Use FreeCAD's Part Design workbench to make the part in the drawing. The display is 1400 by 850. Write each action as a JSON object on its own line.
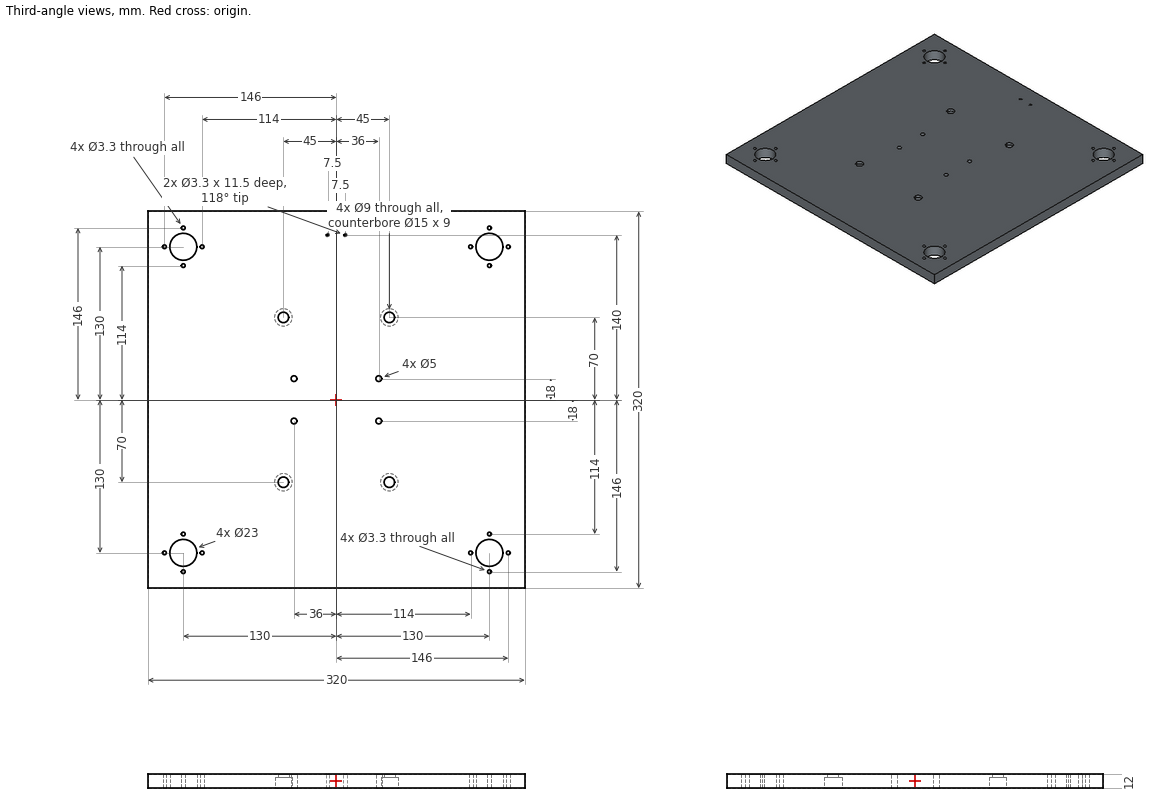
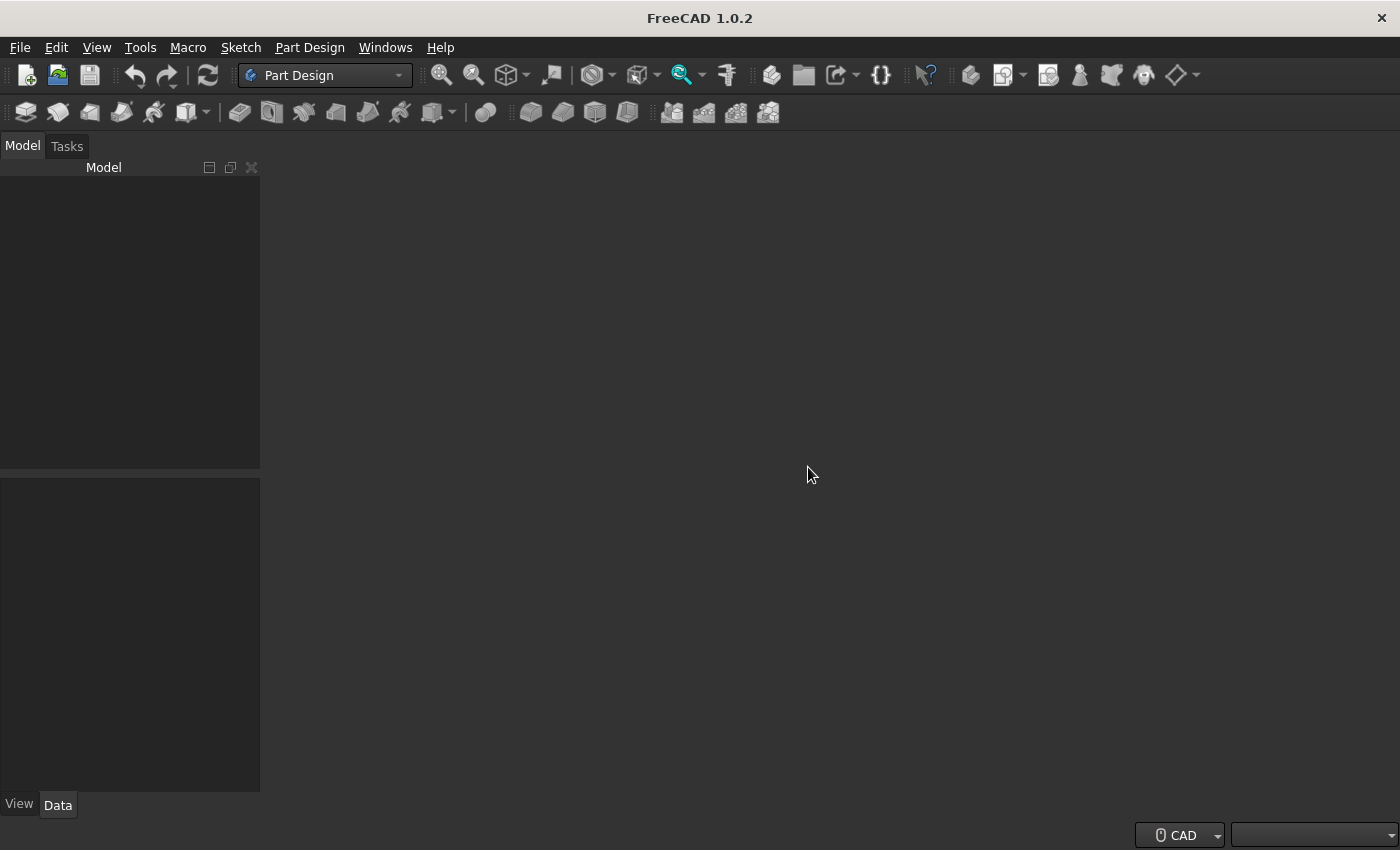
{"action": "left_click", "coordinate": [26, 76]}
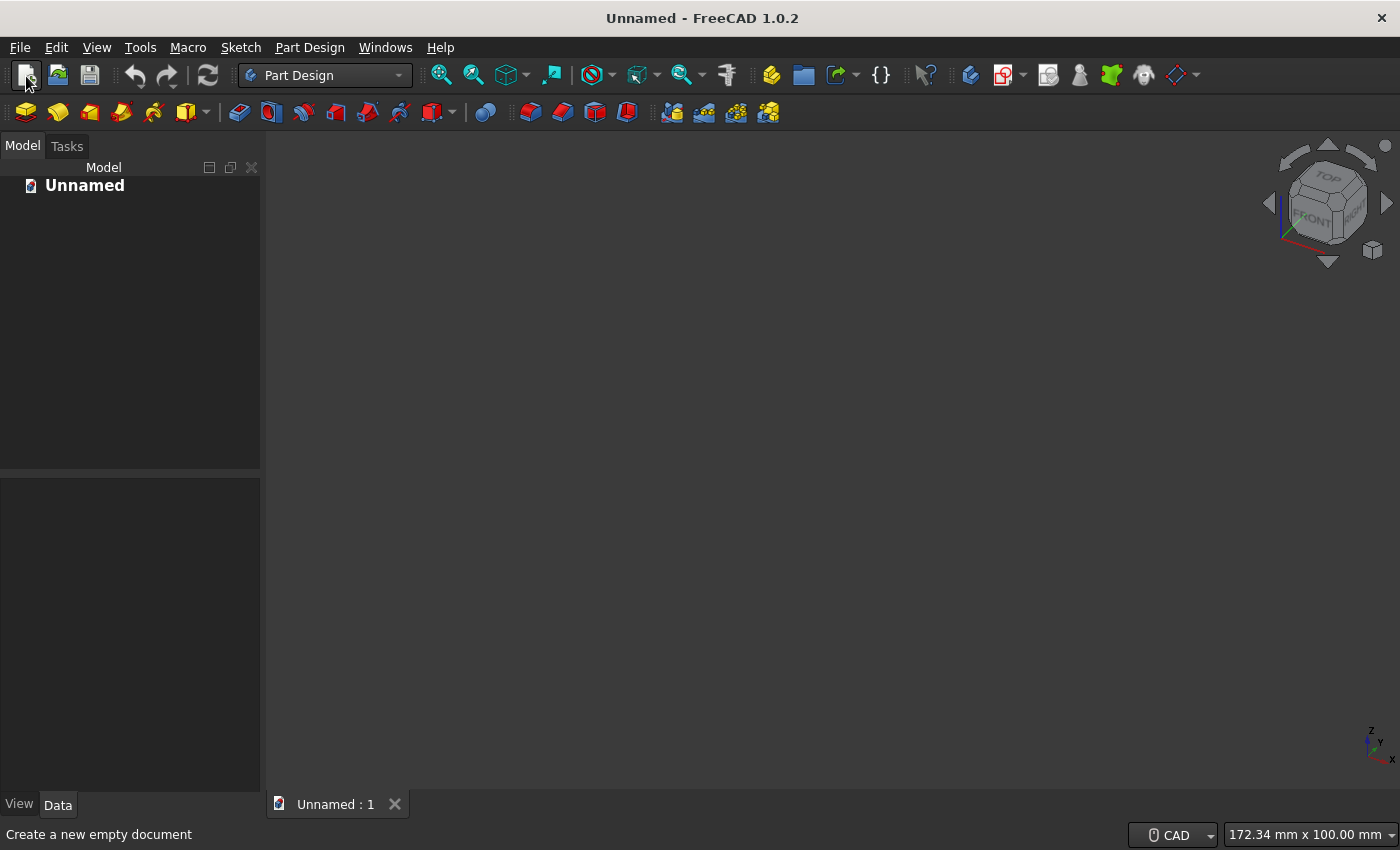
{"action": "left_click", "coordinate": [1004, 76]}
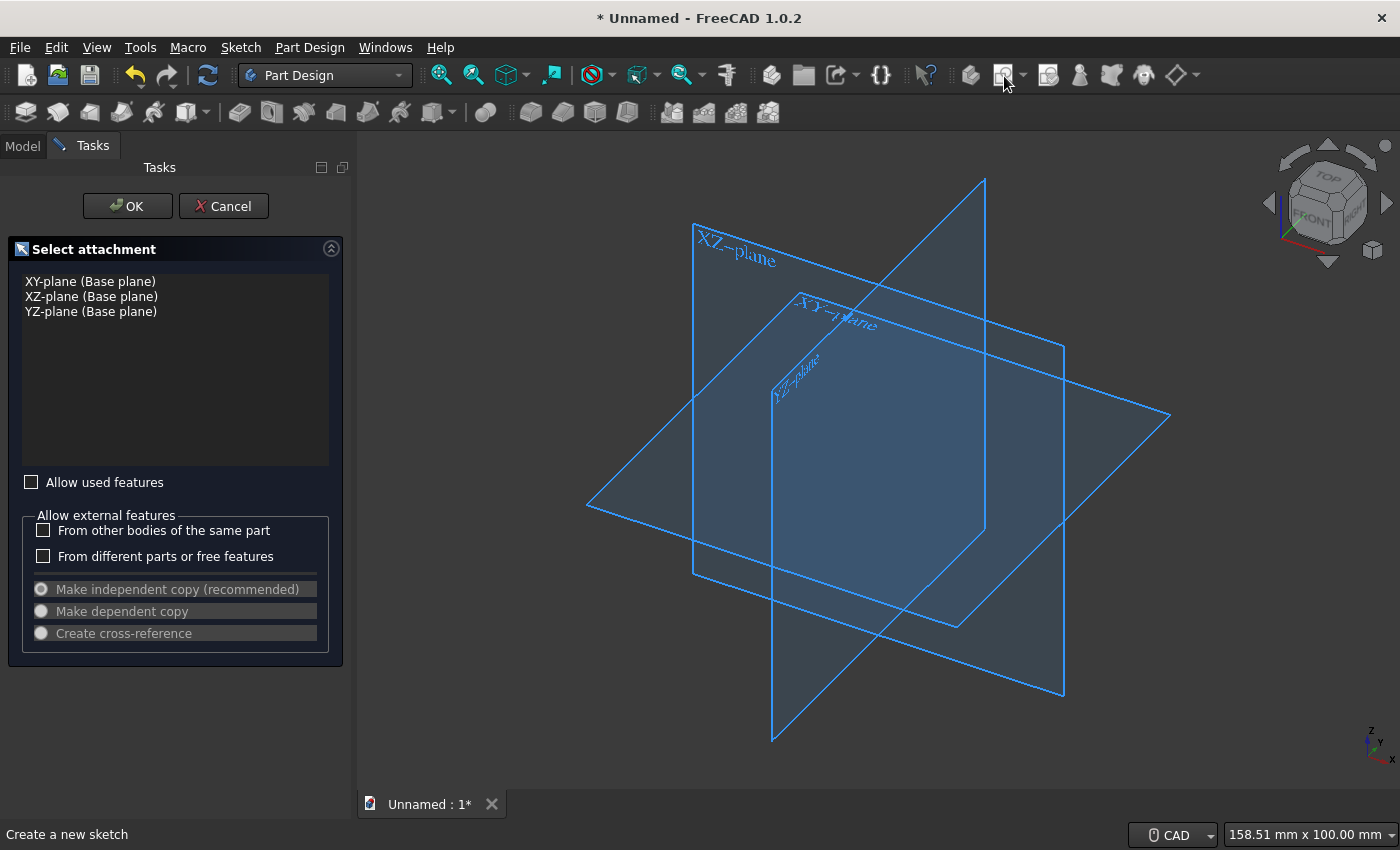
{"action": "left_click", "coordinate": [82, 282]}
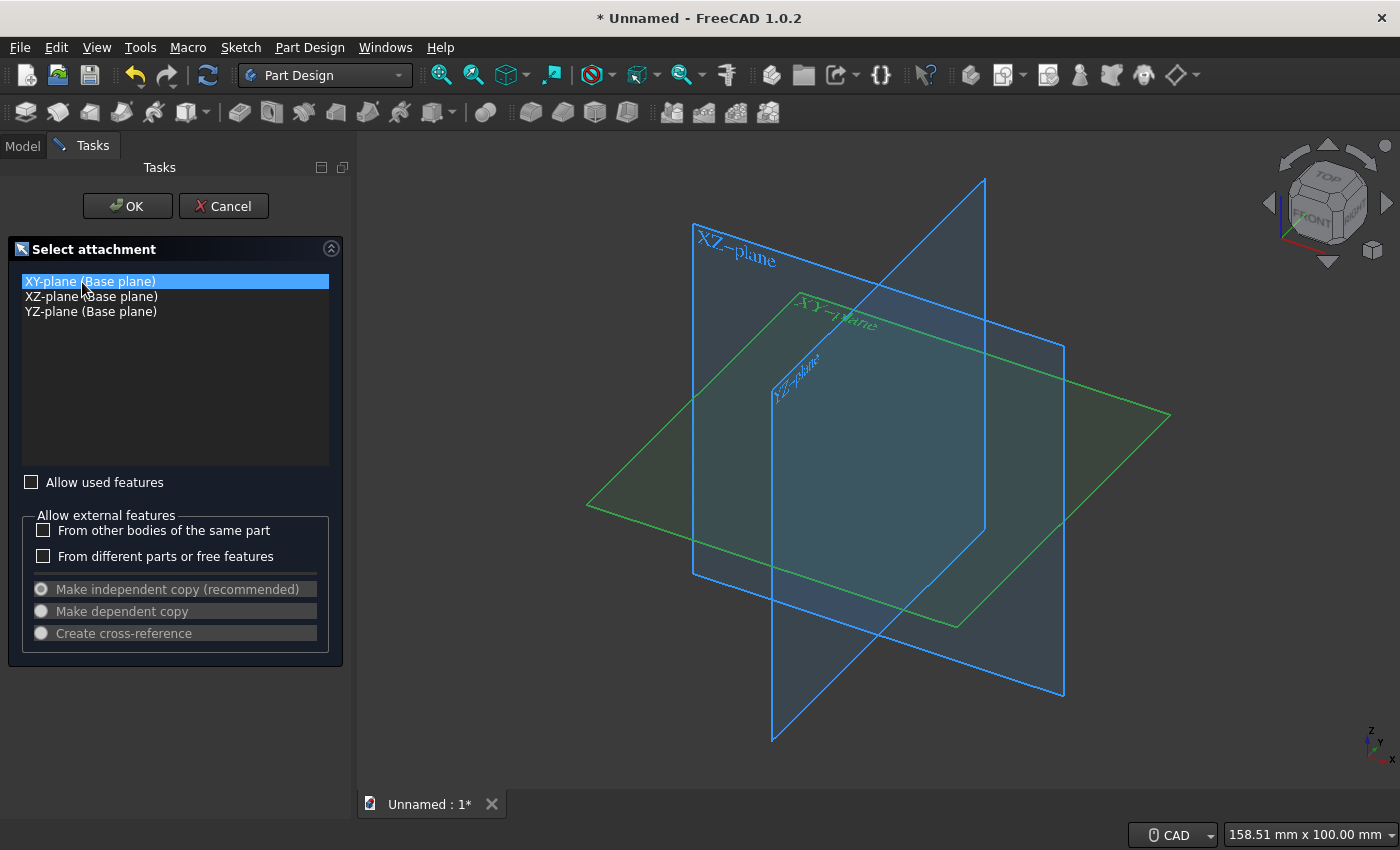
{"action": "left_click", "coordinate": [128, 206]}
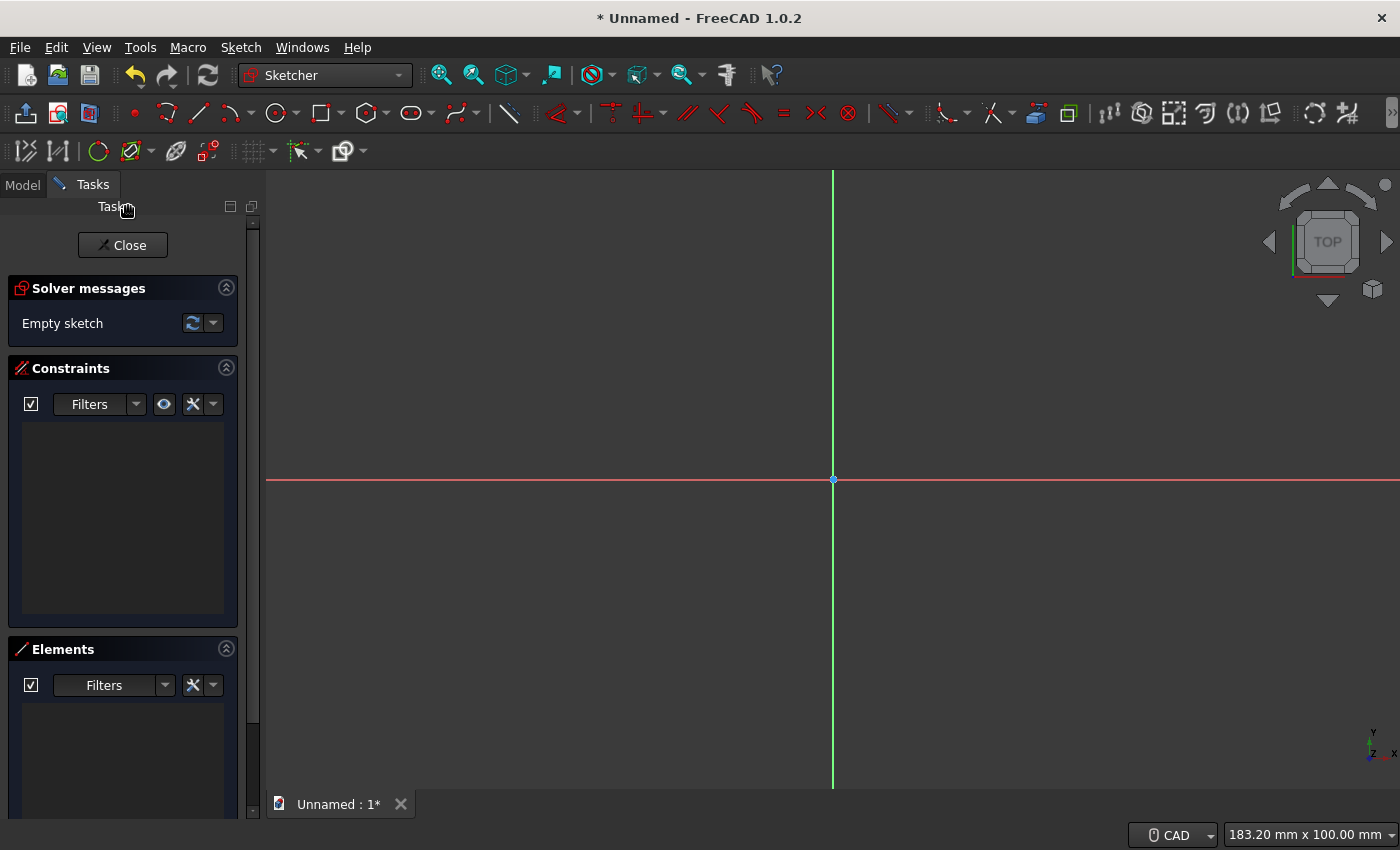
{"action": "scroll", "coordinate": [747, 480], "scroll_direction": "down", "scroll_amount": 8}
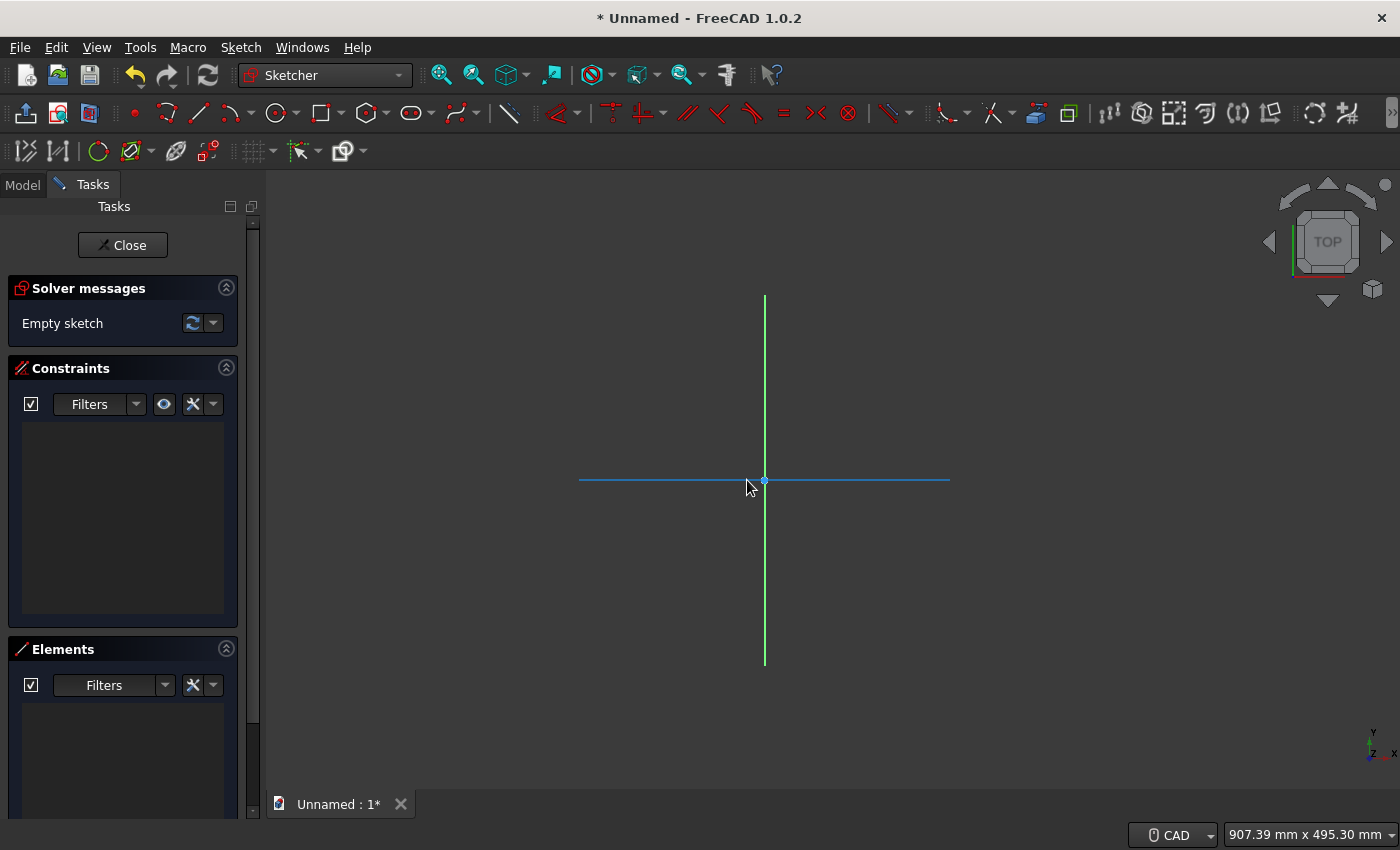
{"action": "key", "text": "g v"}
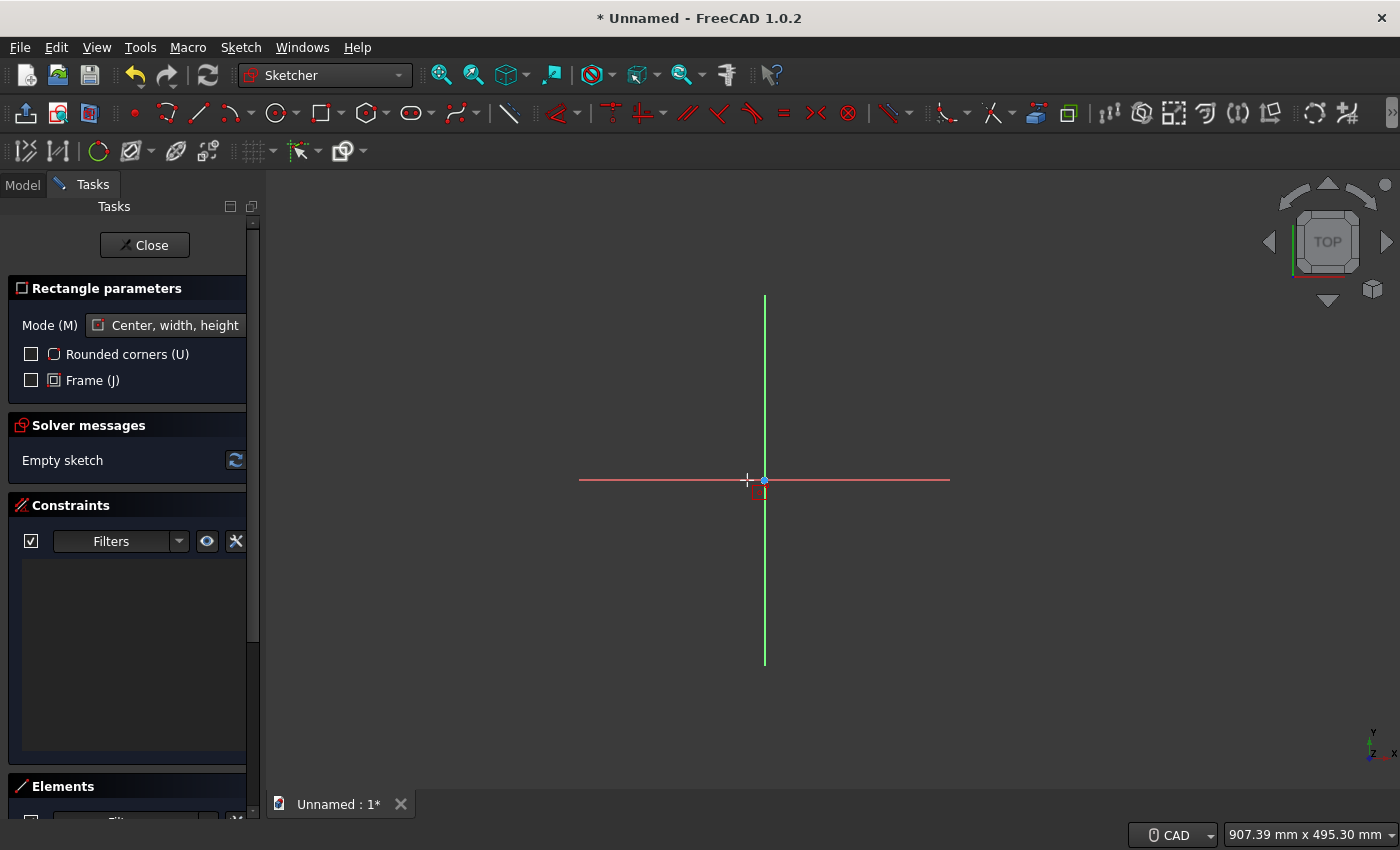
{"action": "left_click", "coordinate": [765, 480]}
{"action": "mouse_move", "coordinate": [965, 280]}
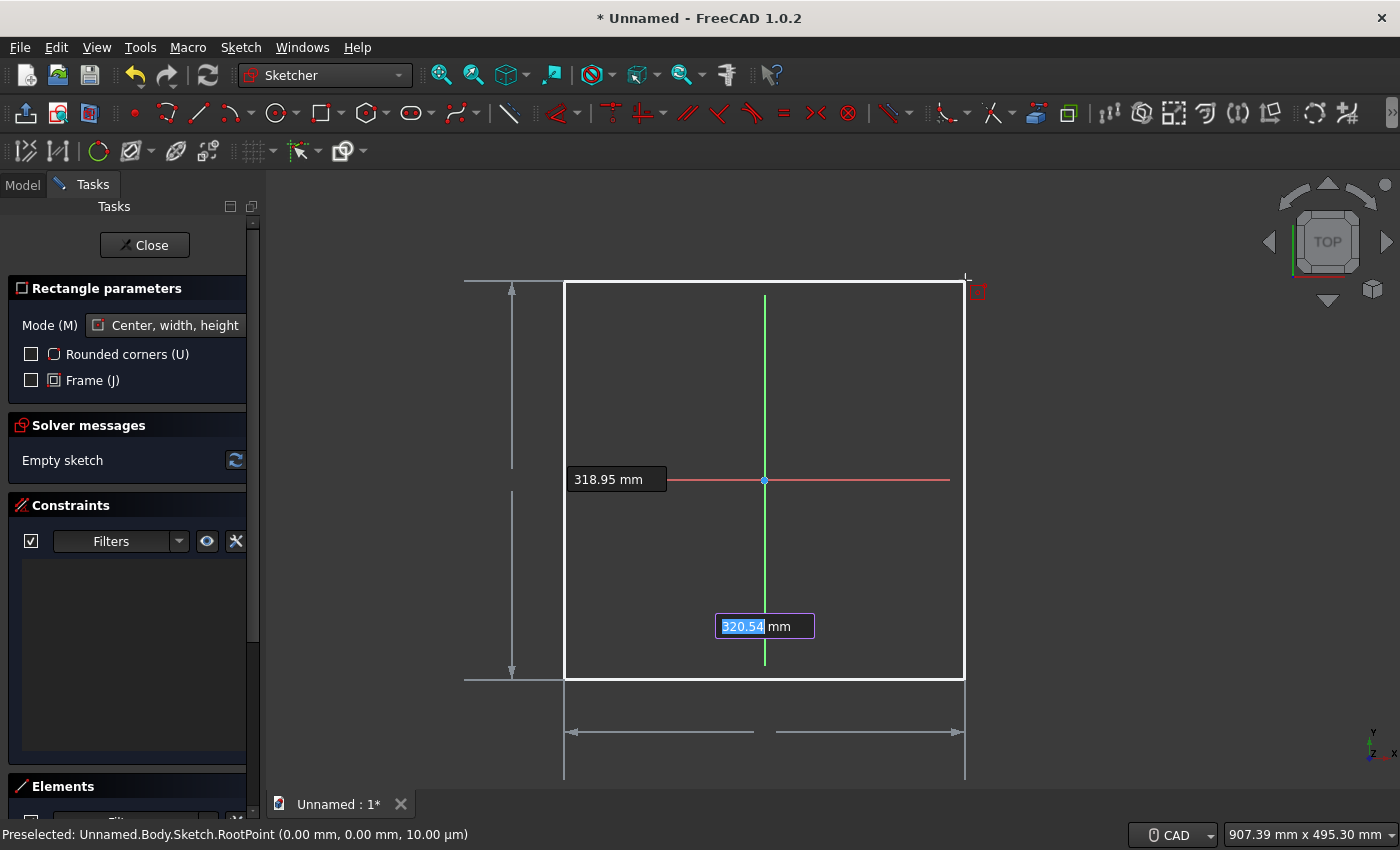
{"action": "type", "text": "320"}
{"action": "key", "text": "Tab"}
{"action": "type", "text": "320"}
{"action": "key", "text": "Return"}